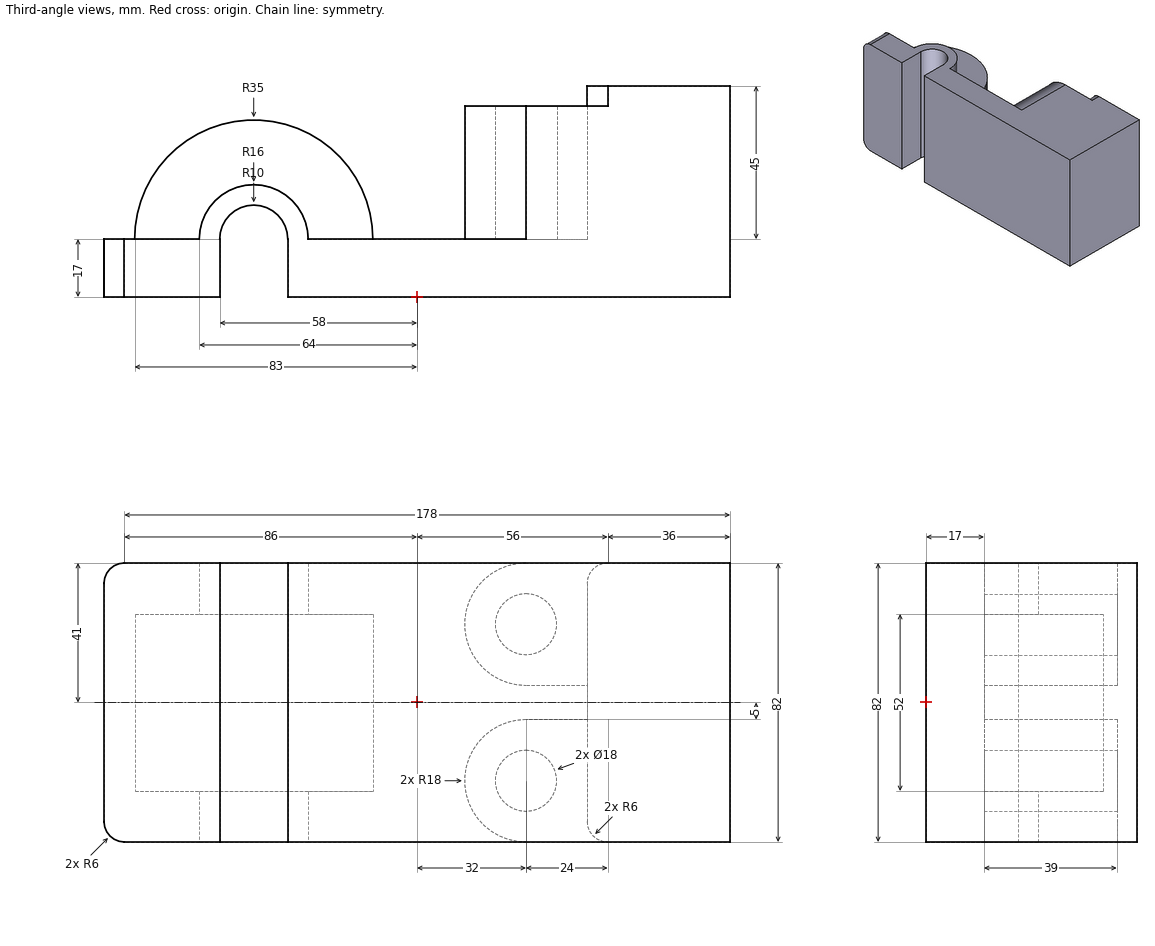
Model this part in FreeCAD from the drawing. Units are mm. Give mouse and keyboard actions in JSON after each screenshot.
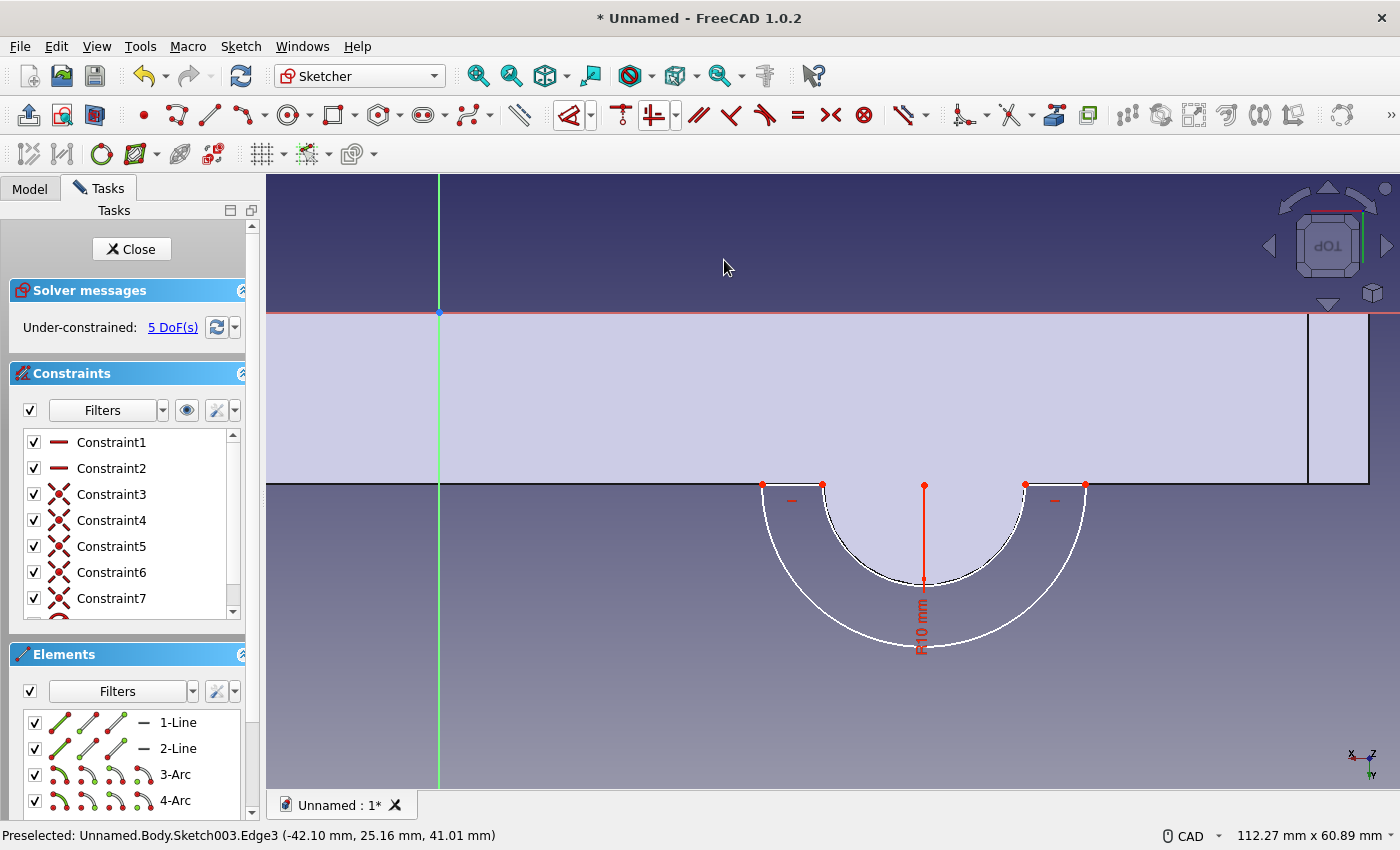
{"action": "left_click", "coordinate": [829, 616]}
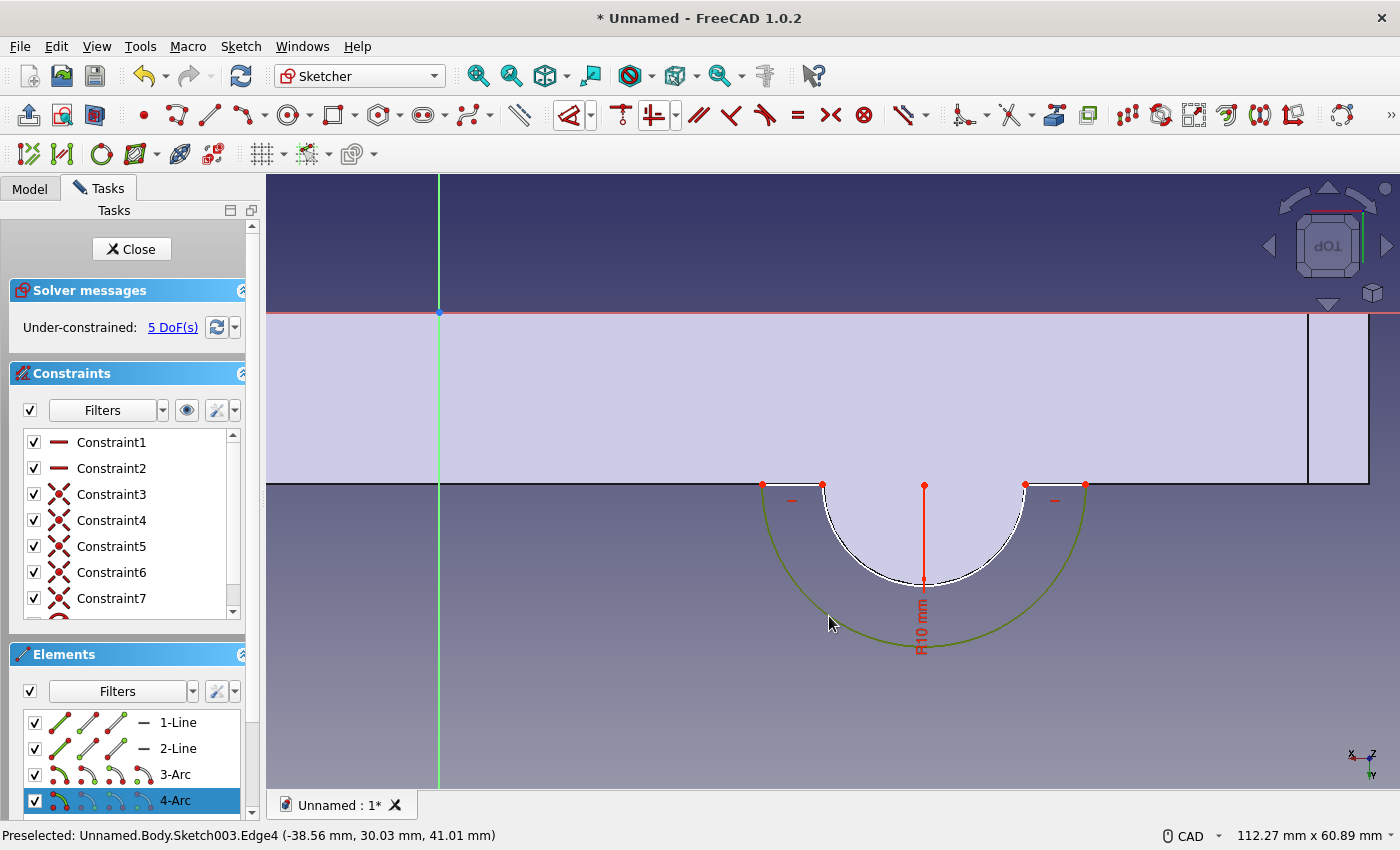
{"action": "key", "text": "k r"}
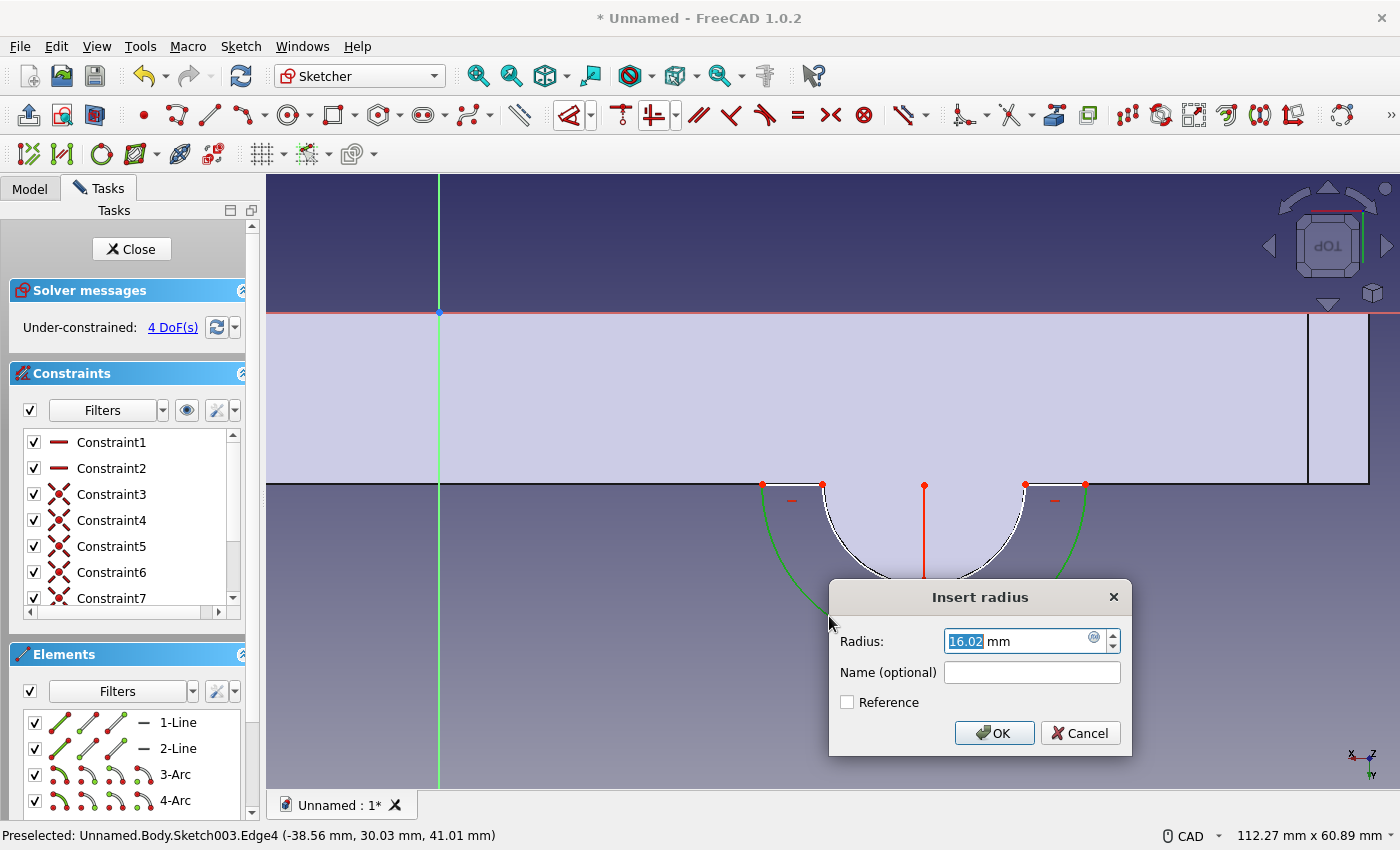
{"action": "type", "text": "16"}
{"action": "key", "text": "Return"}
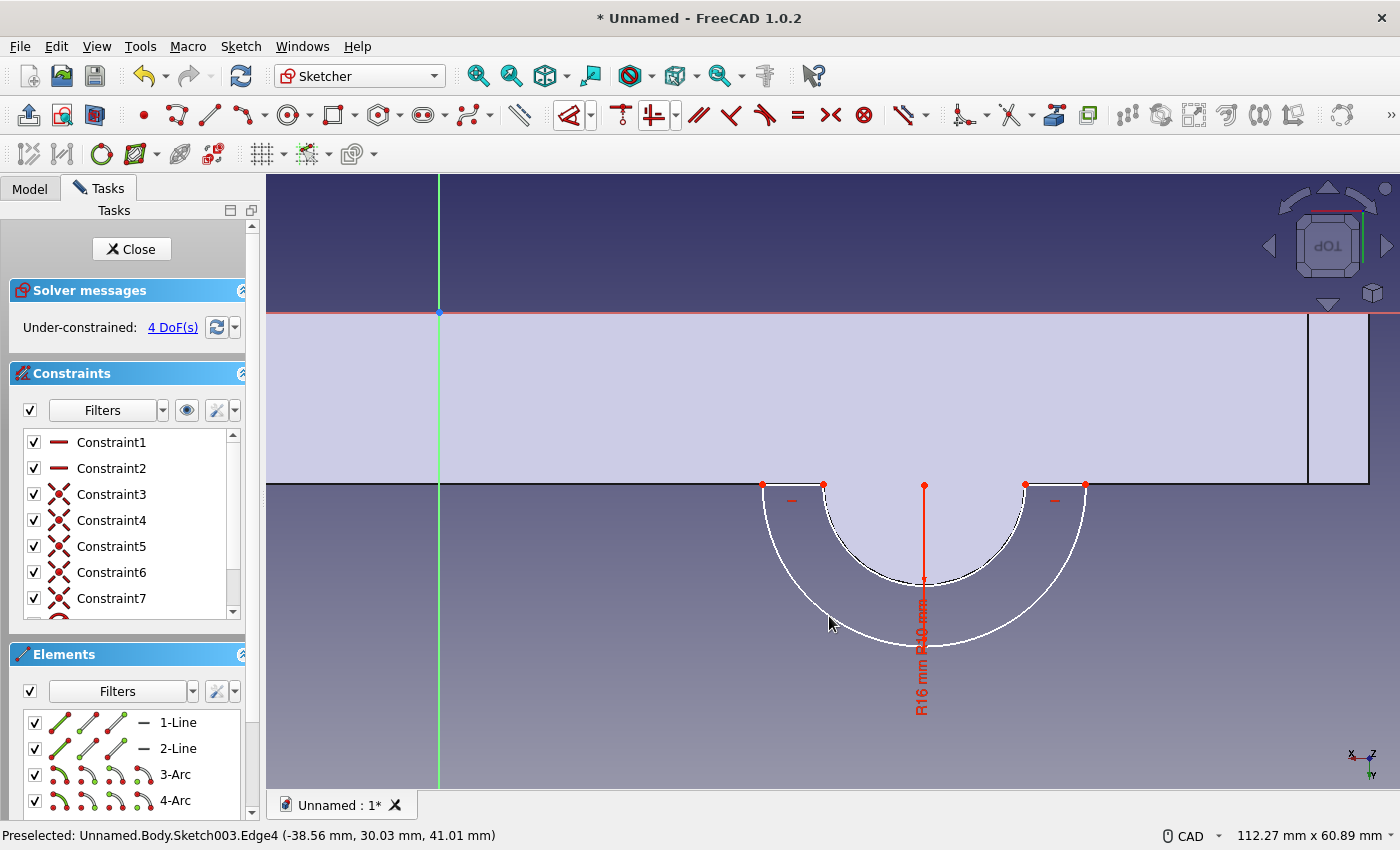
{"action": "left_click", "coordinate": [1086, 485]}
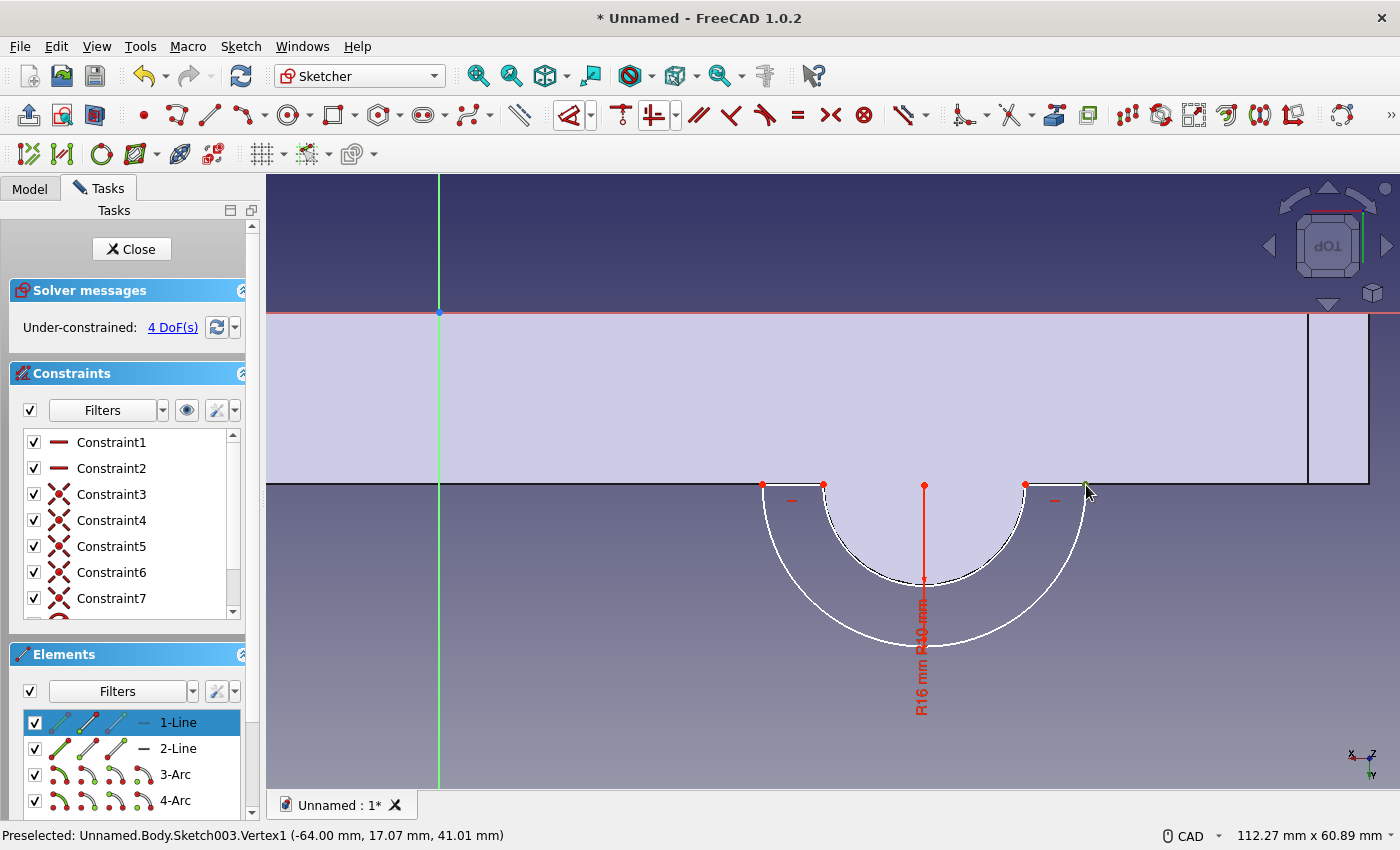
{"action": "left_click", "coordinate": [590, 116]}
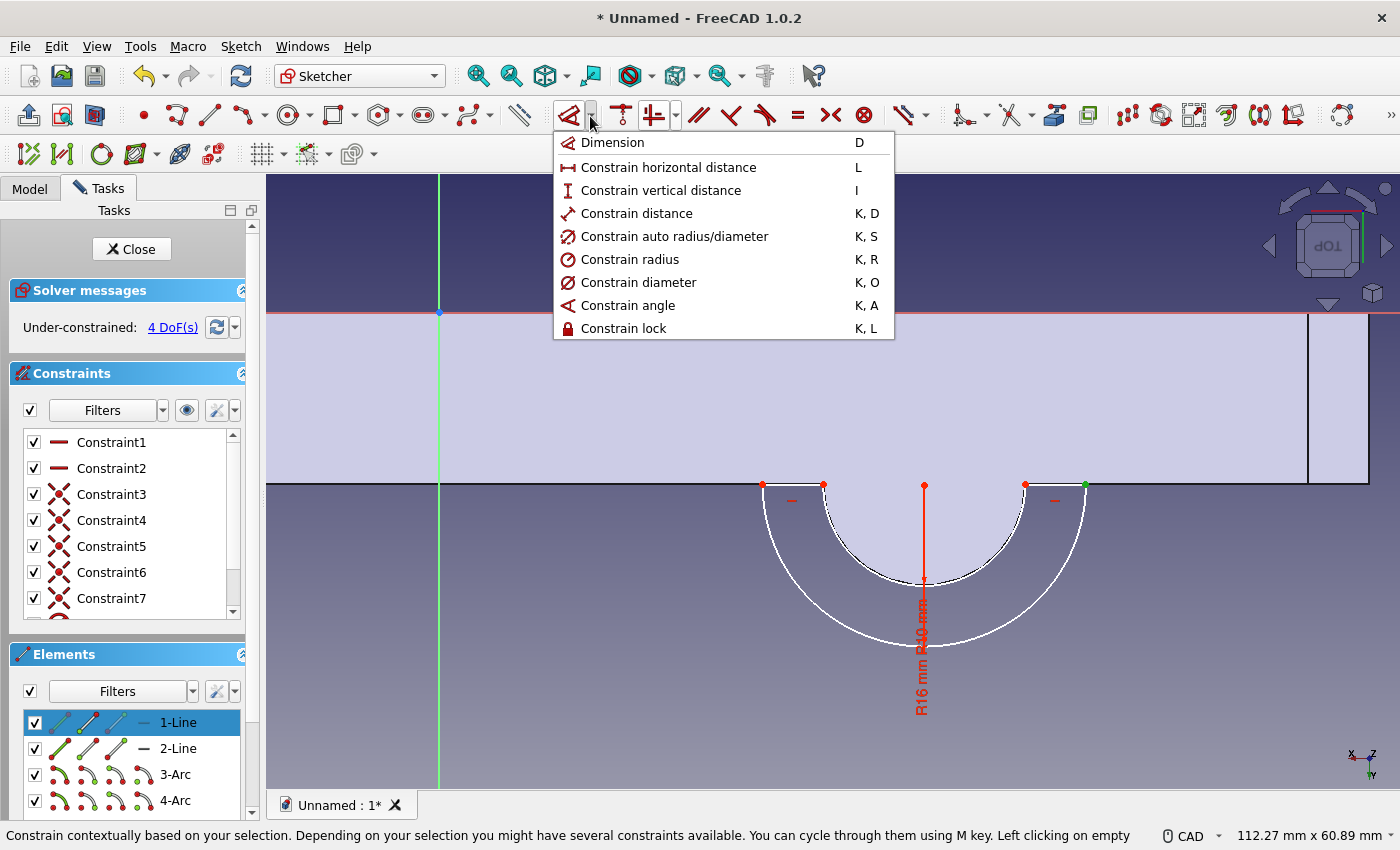
{"action": "left_click", "coordinate": [724, 168]}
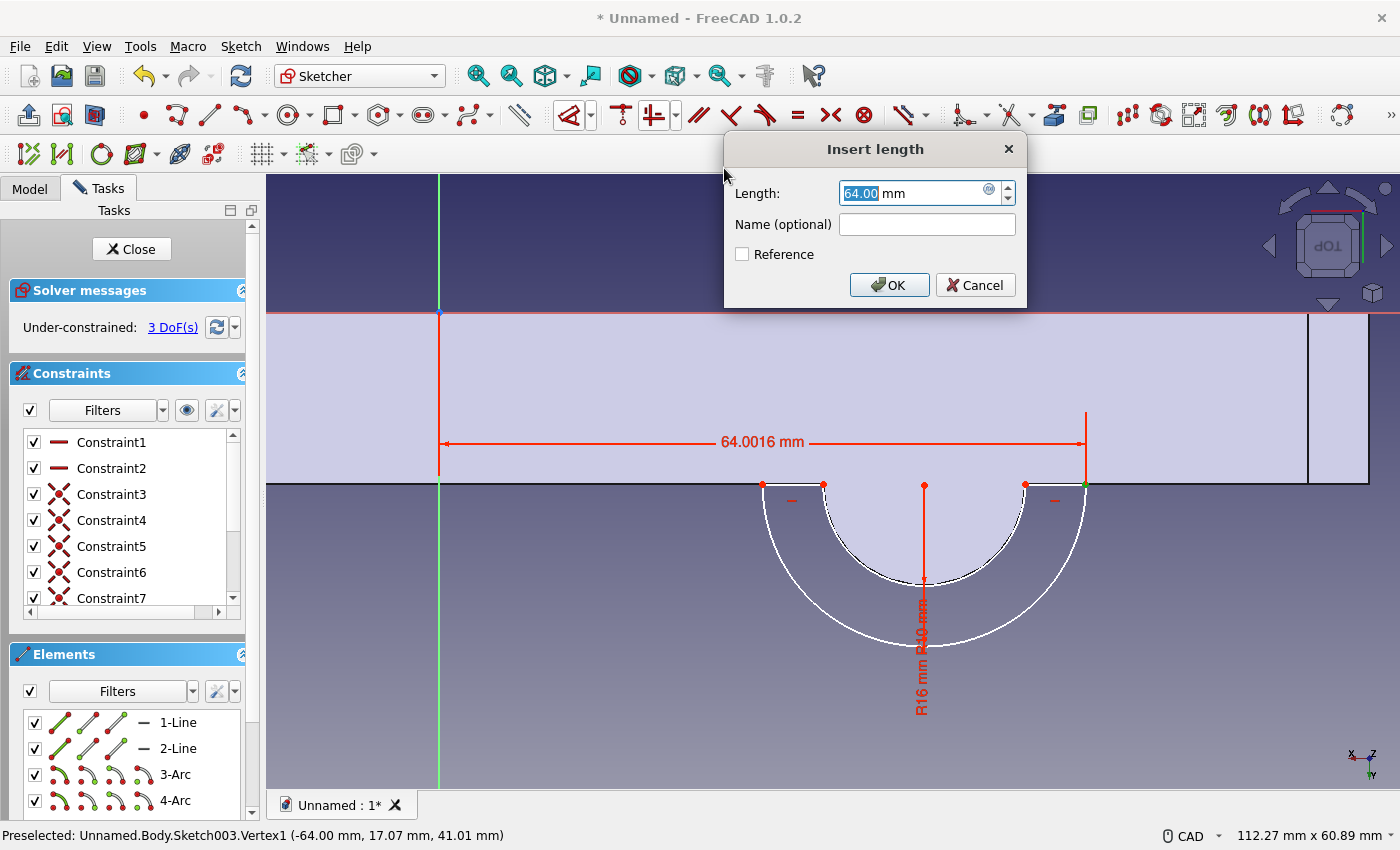
{"action": "type", "text": "64"}
{"action": "key", "text": "Return"}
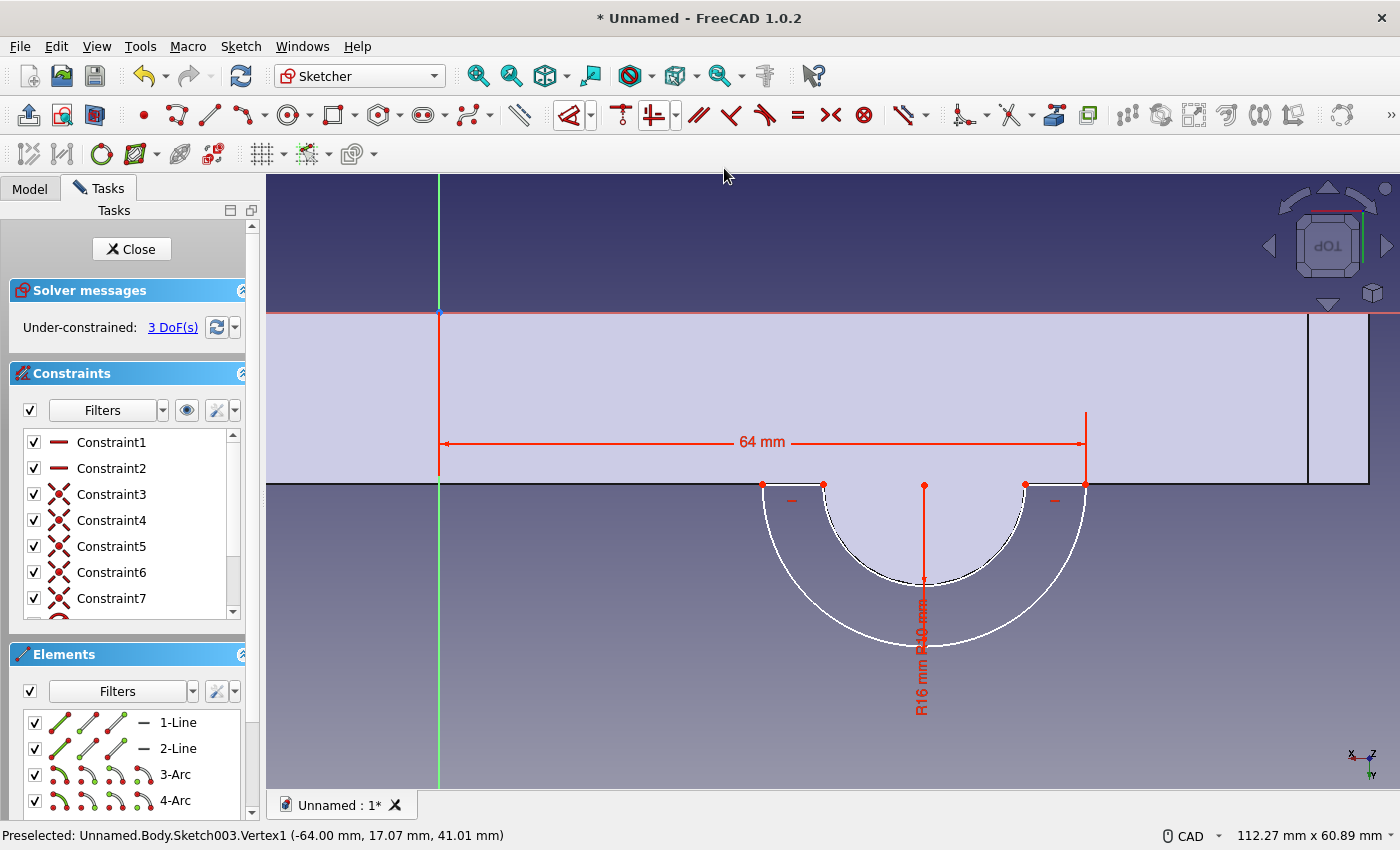
{"action": "left_click", "coordinate": [1086, 485]}